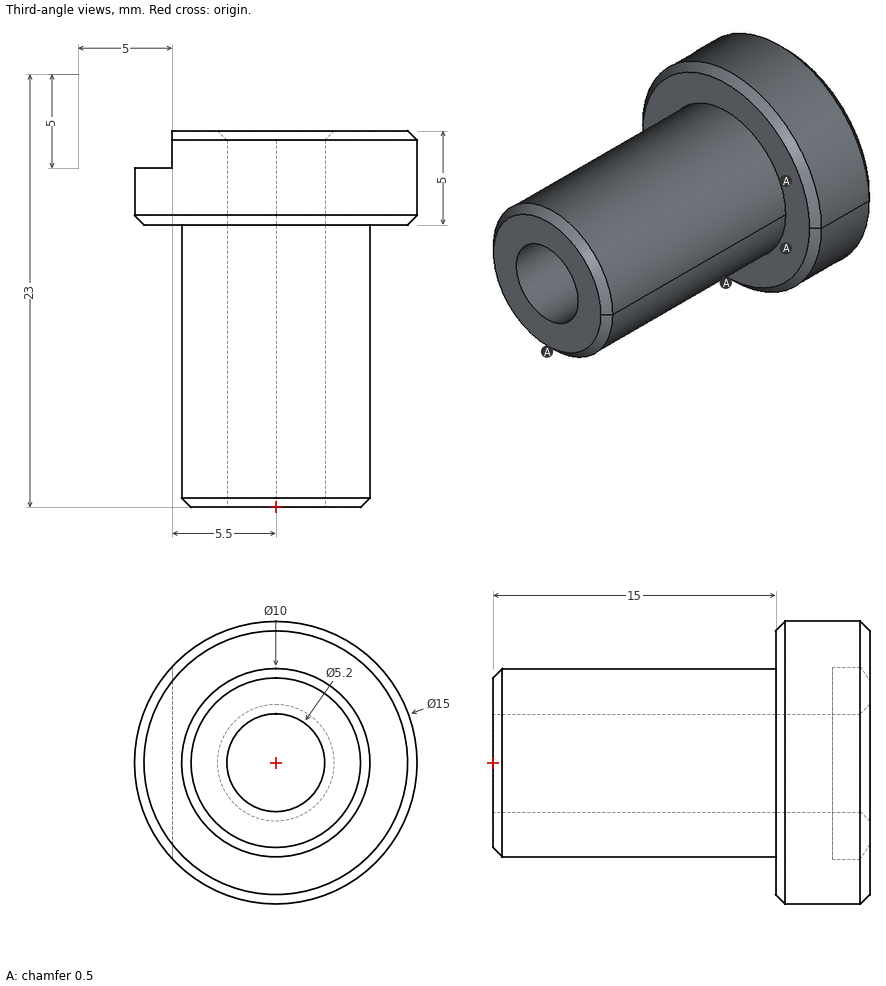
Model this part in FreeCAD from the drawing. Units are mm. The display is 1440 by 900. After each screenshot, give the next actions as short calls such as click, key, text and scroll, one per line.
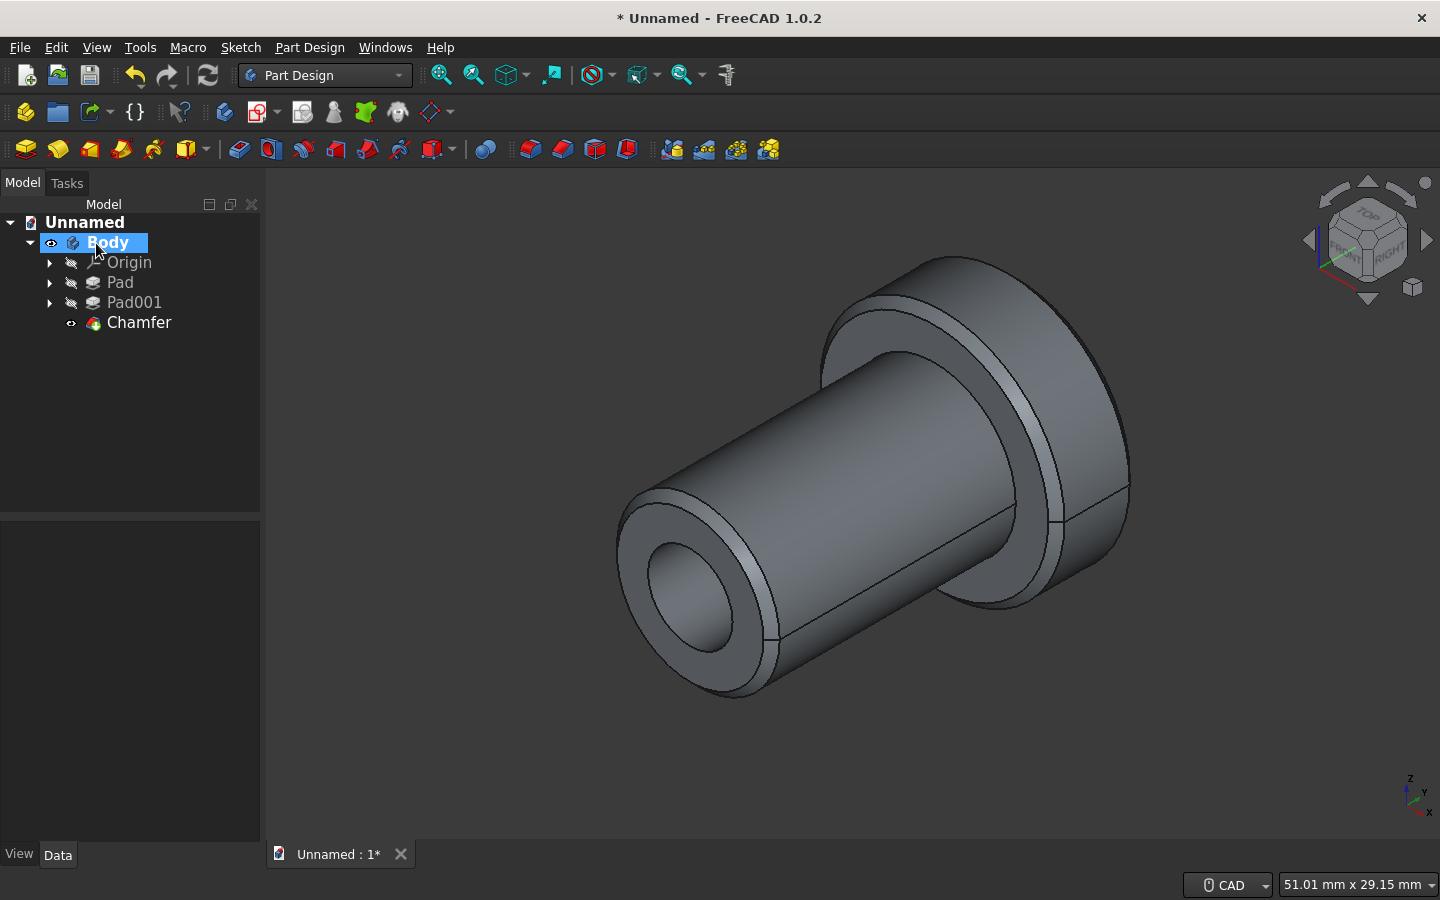
click(258, 112)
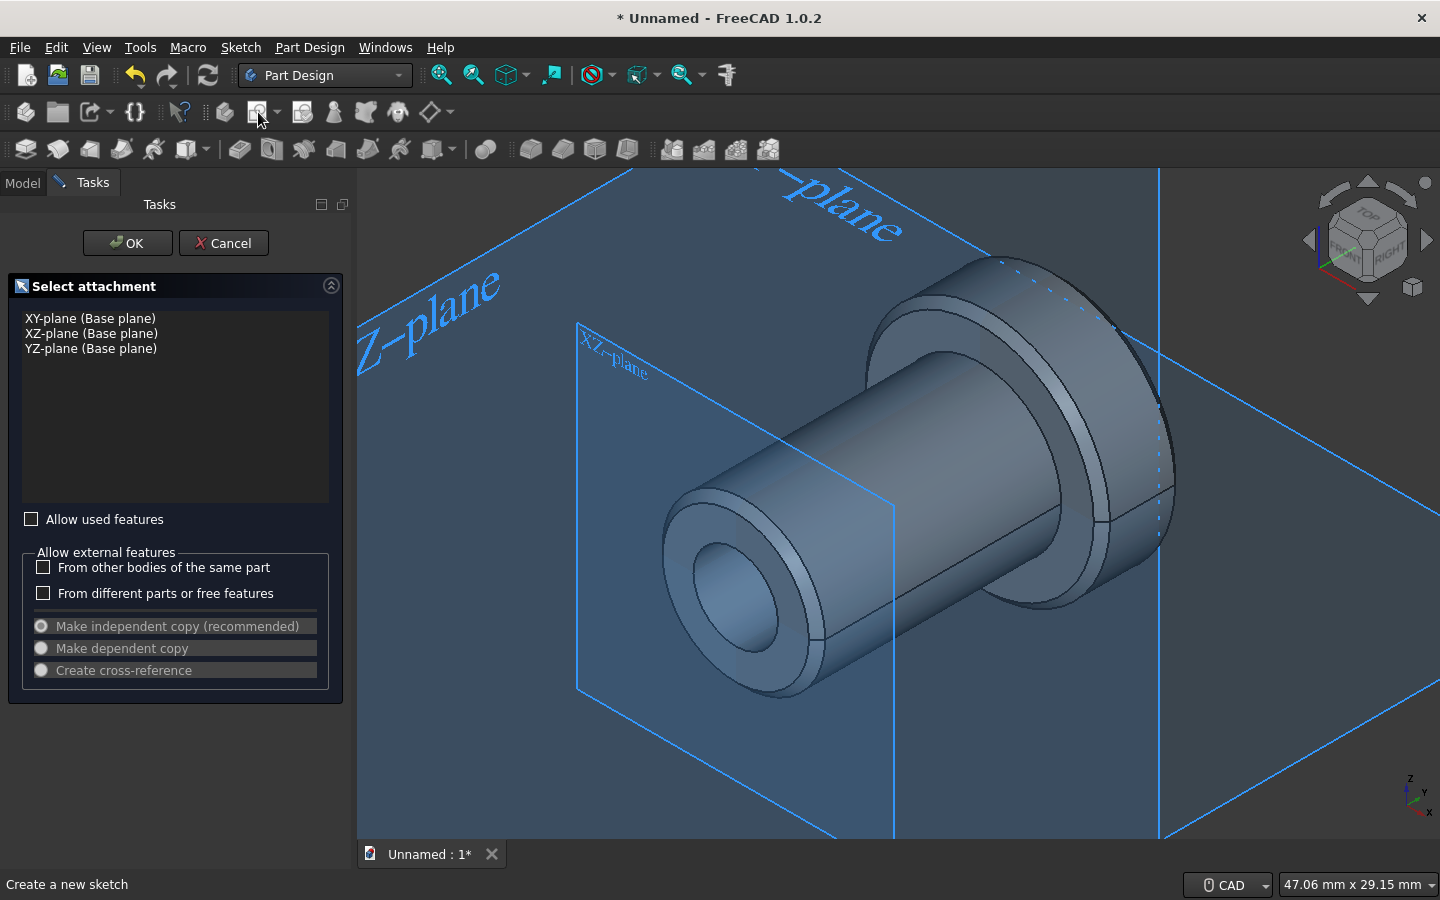
click(82, 318)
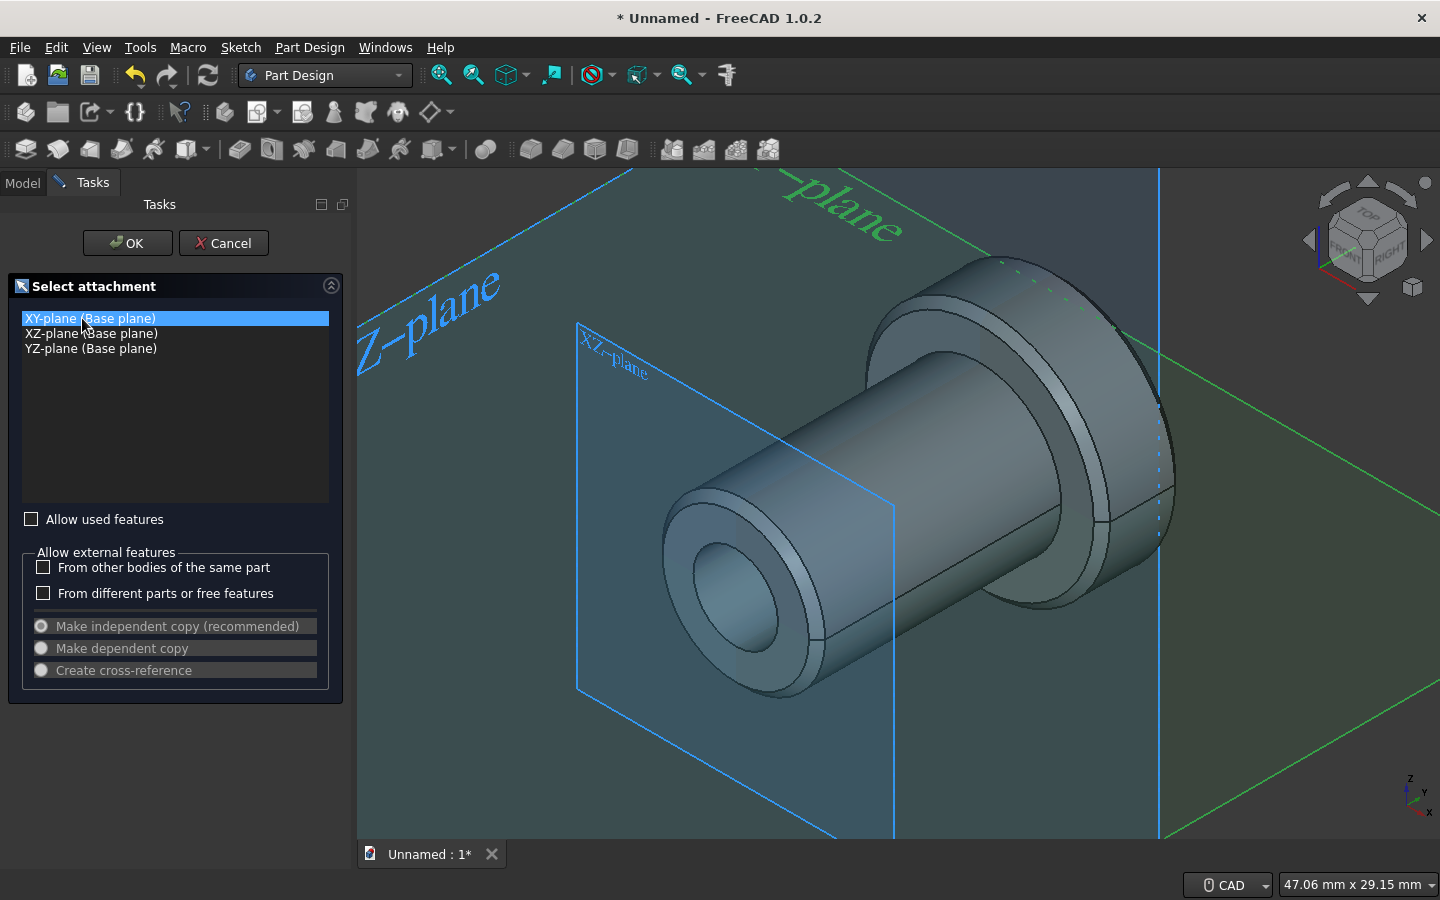
click(128, 243)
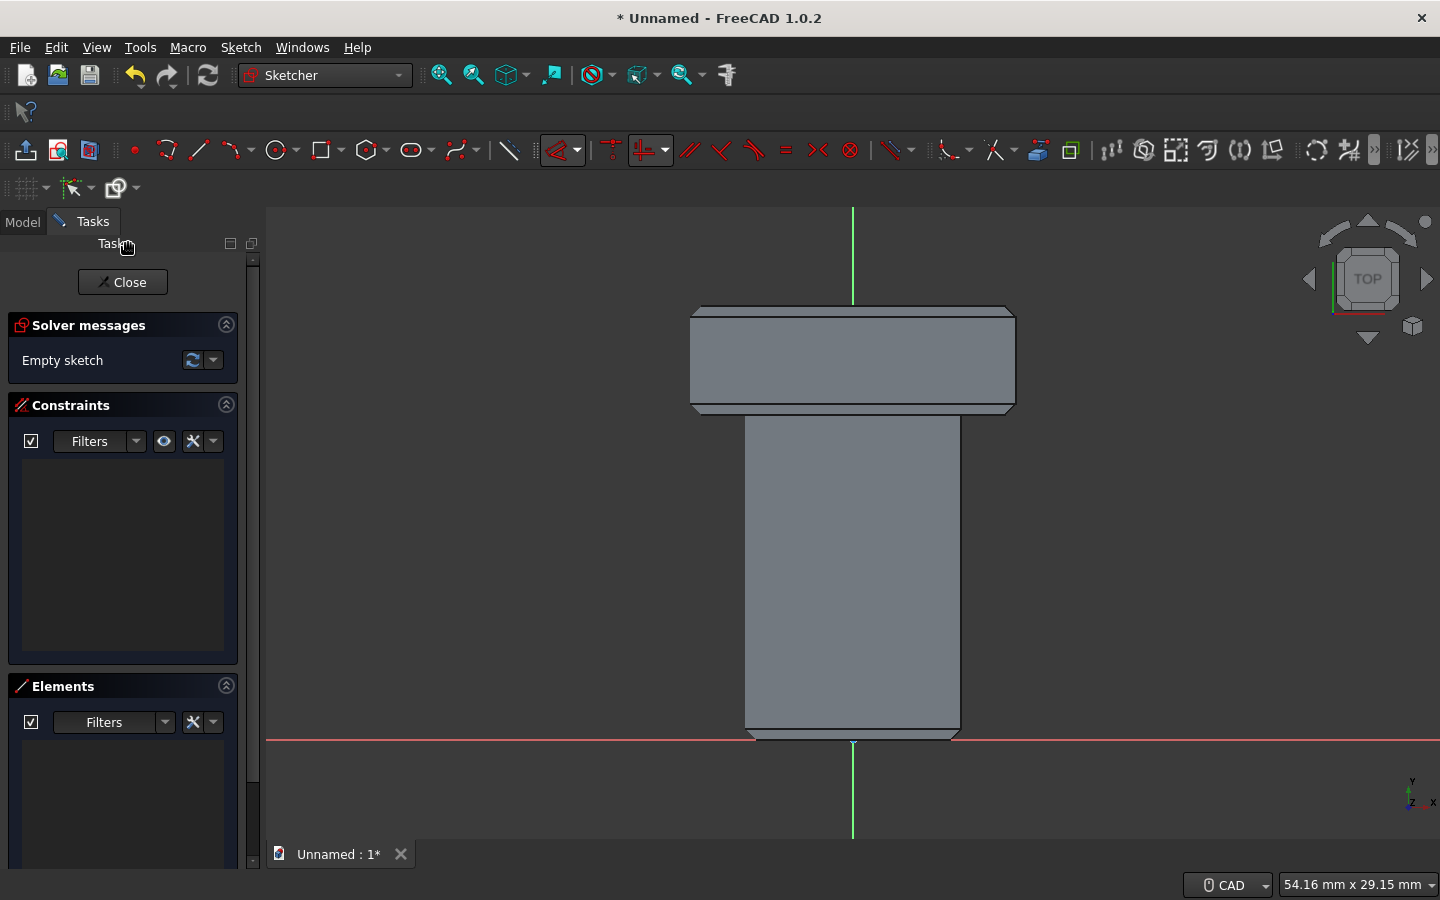
click(90, 150)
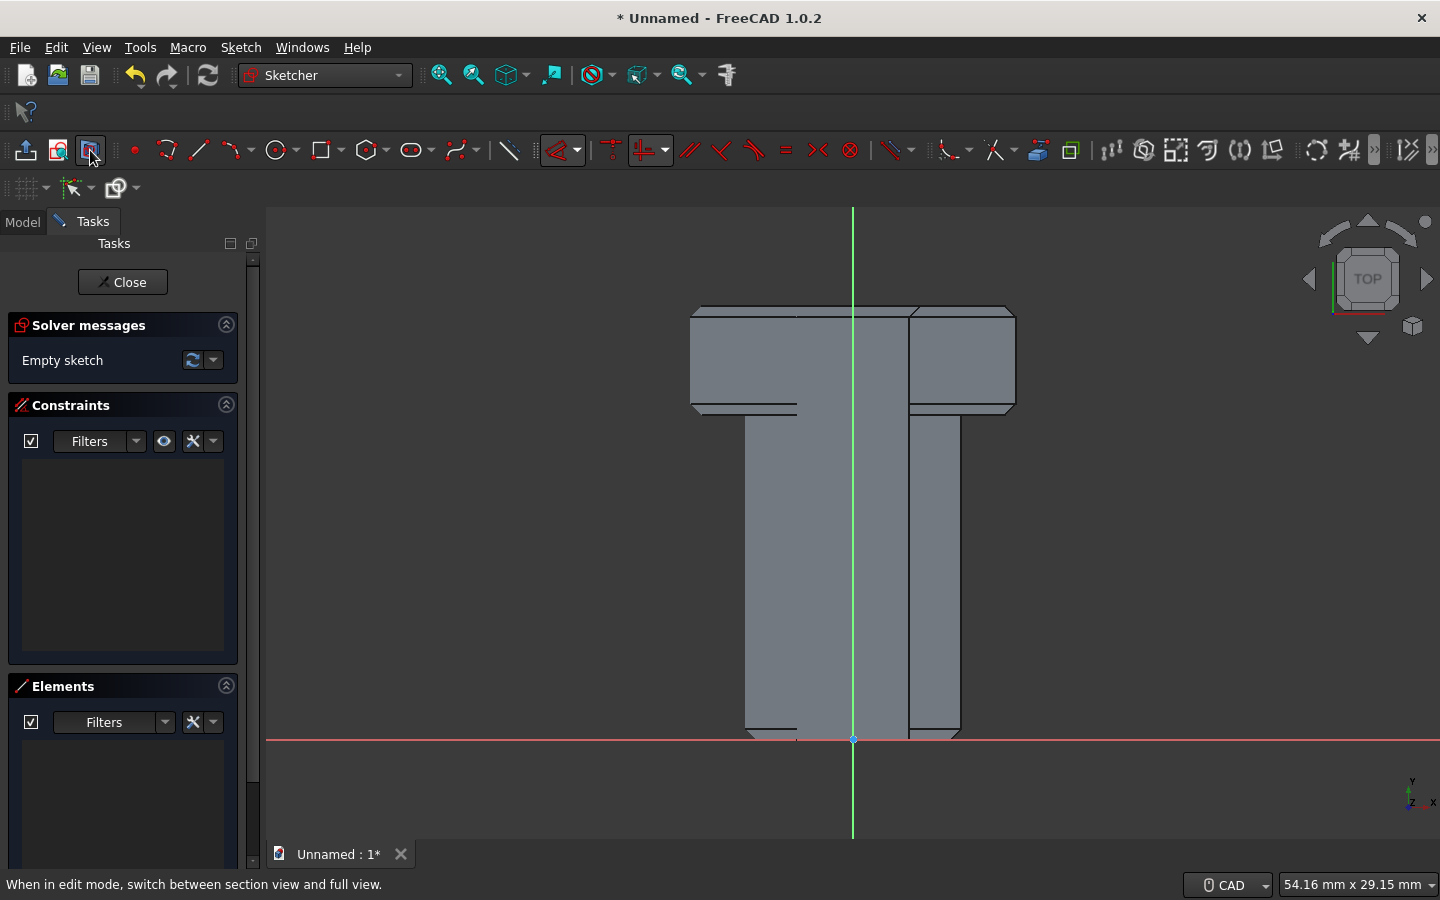
scroll(645, 235, up, 7)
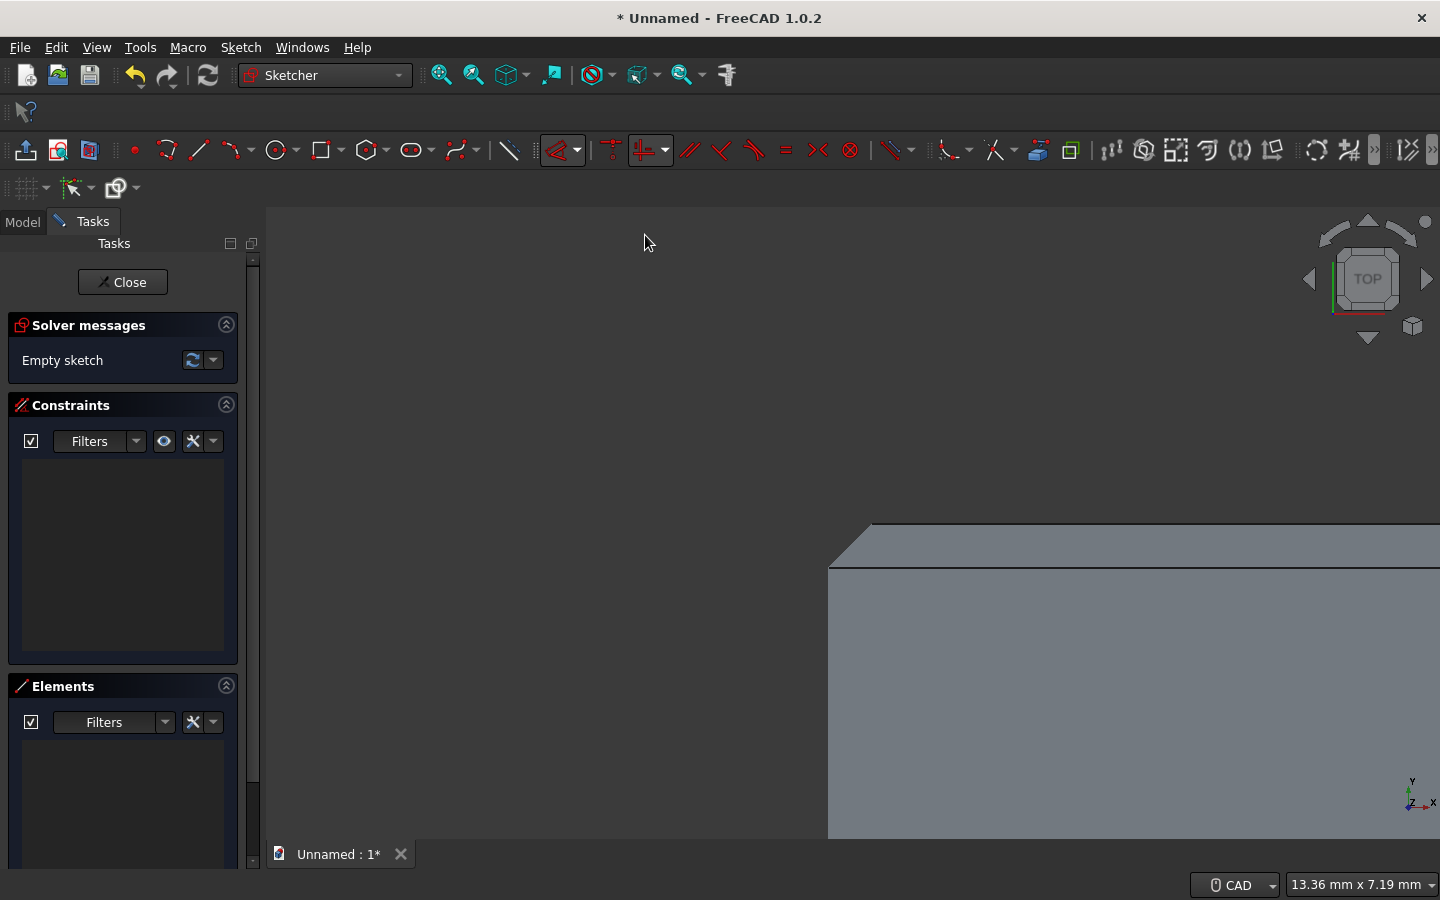
scroll(786, 718, down, 1)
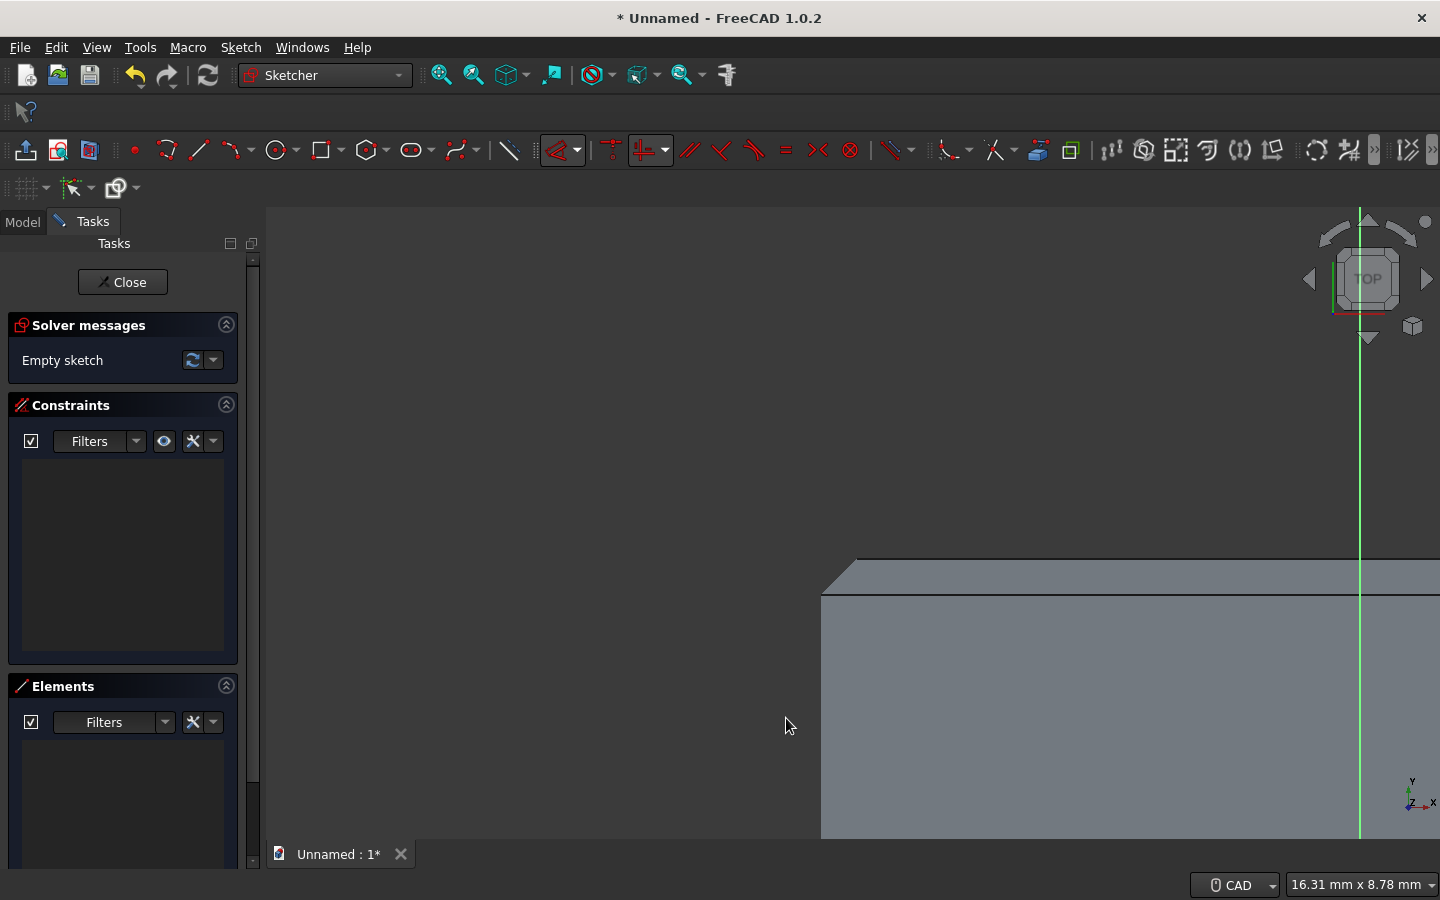
click(322, 150)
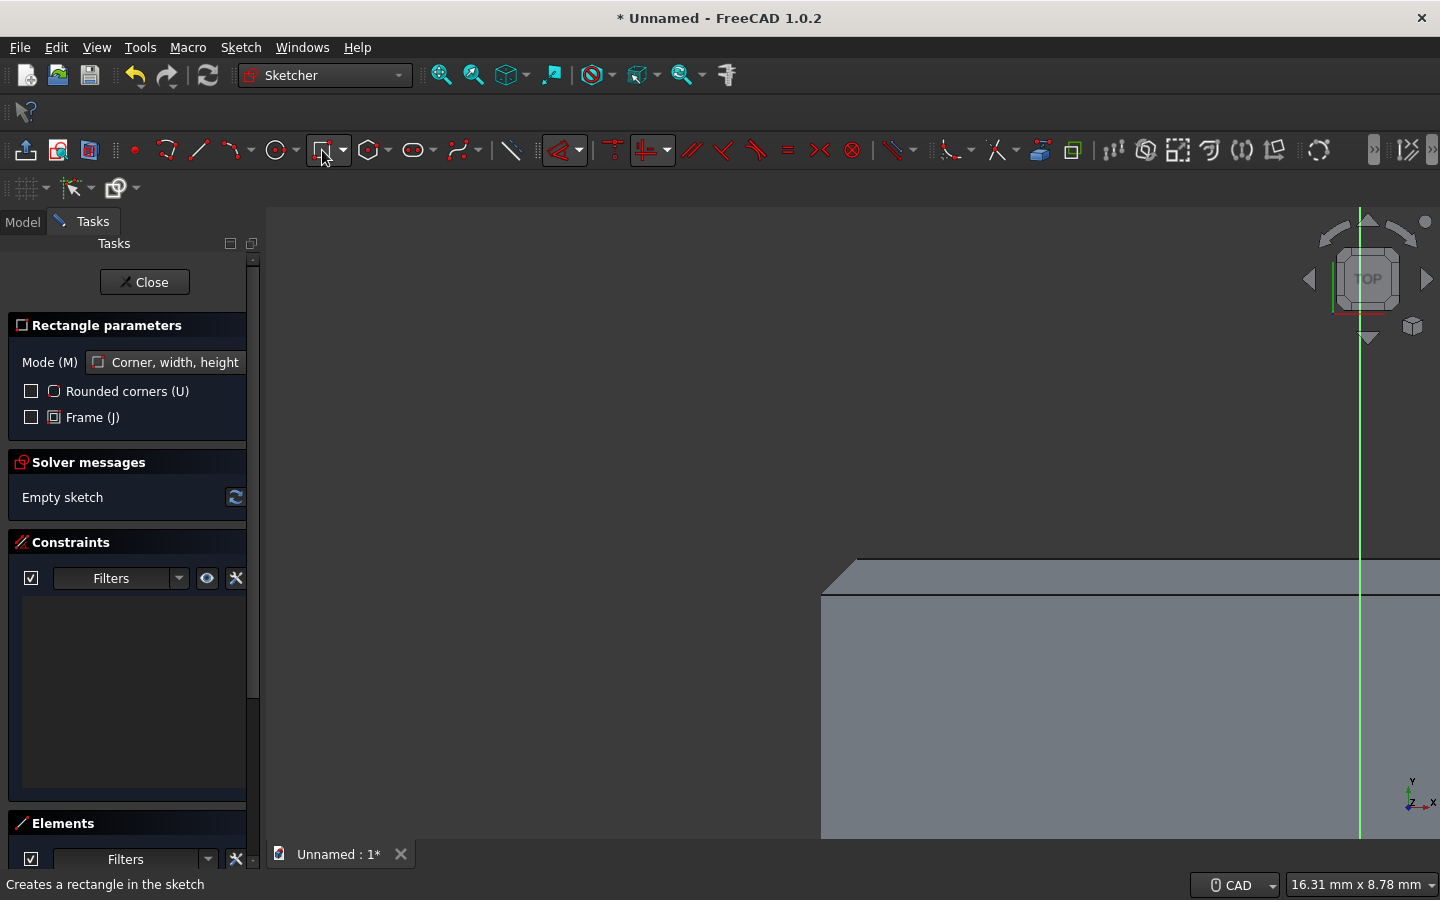
click(605, 343)
click(965, 703)
key(Escape)